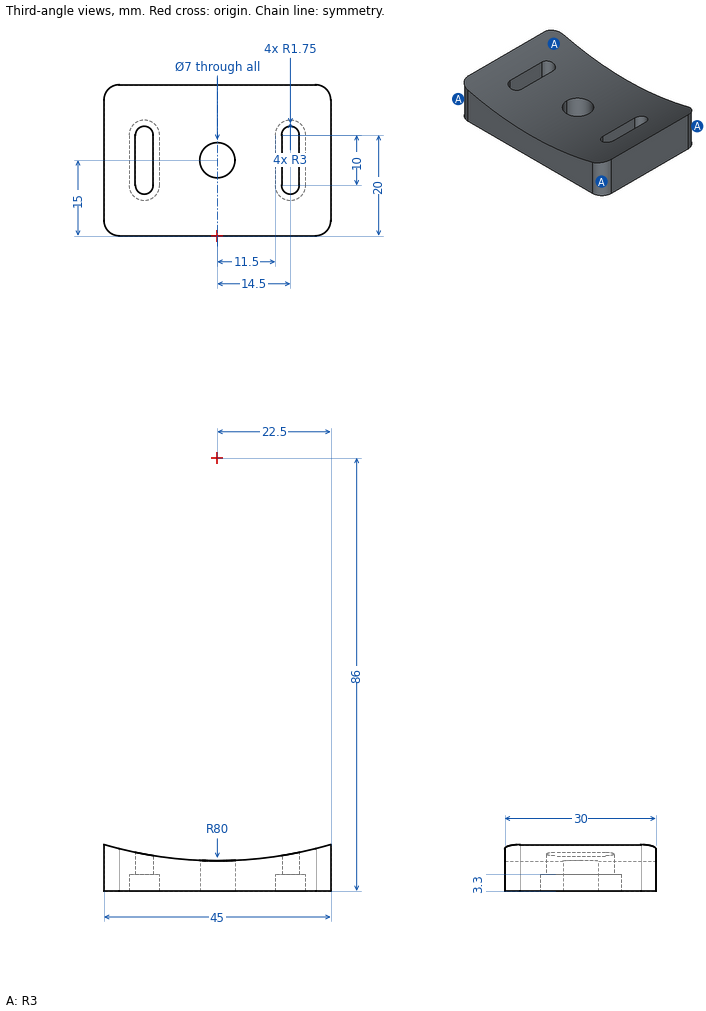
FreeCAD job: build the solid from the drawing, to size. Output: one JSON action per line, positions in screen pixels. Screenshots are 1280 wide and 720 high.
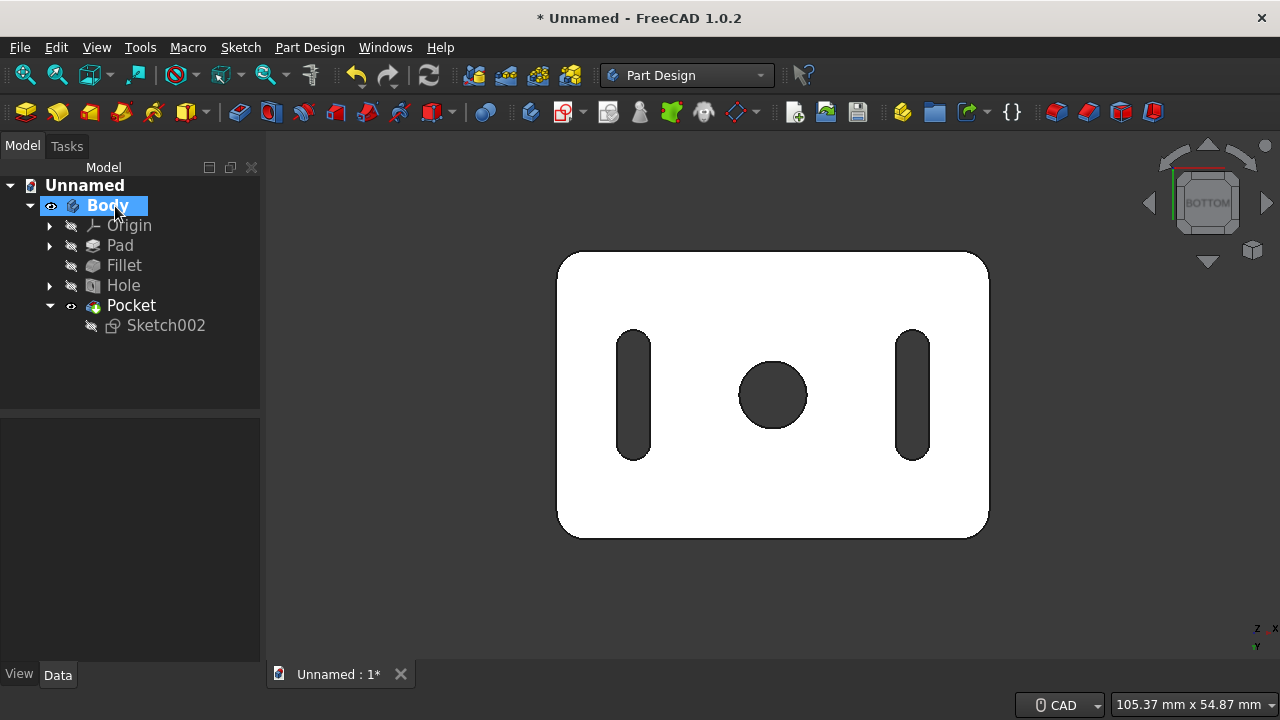
{"action": "left_click", "coordinate": [835, 476]}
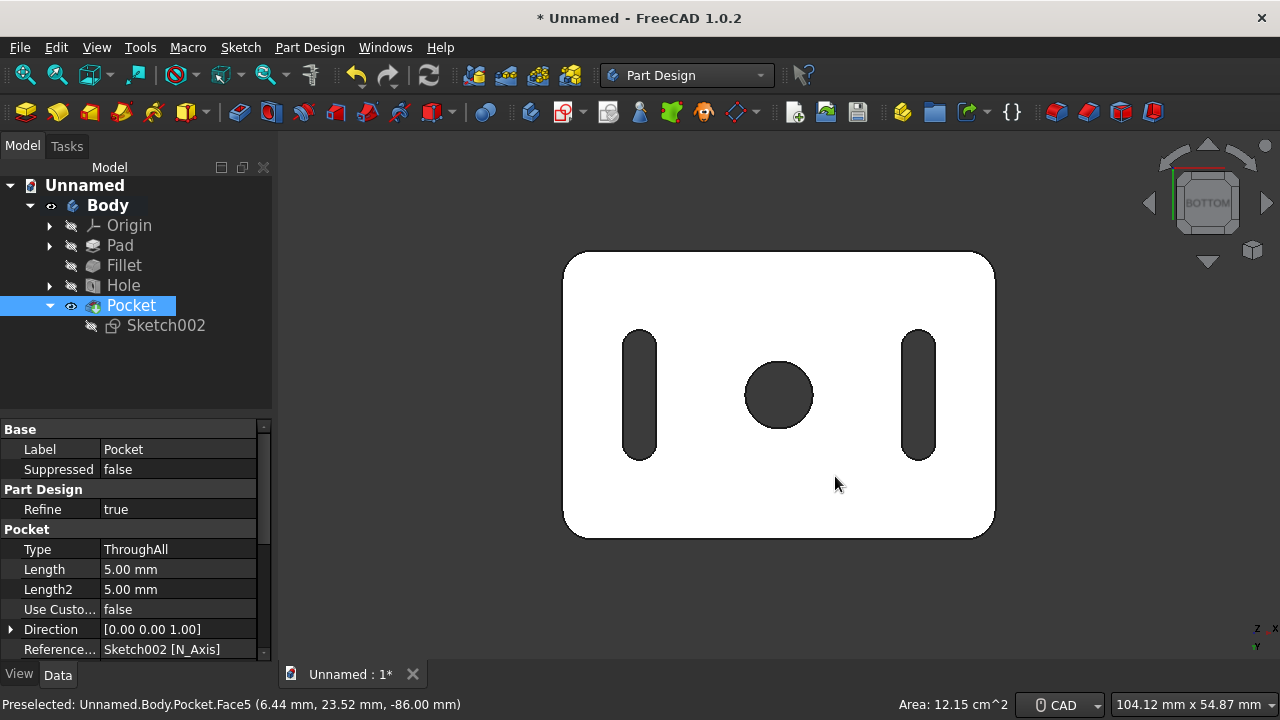
{"action": "left_click", "coordinate": [564, 112]}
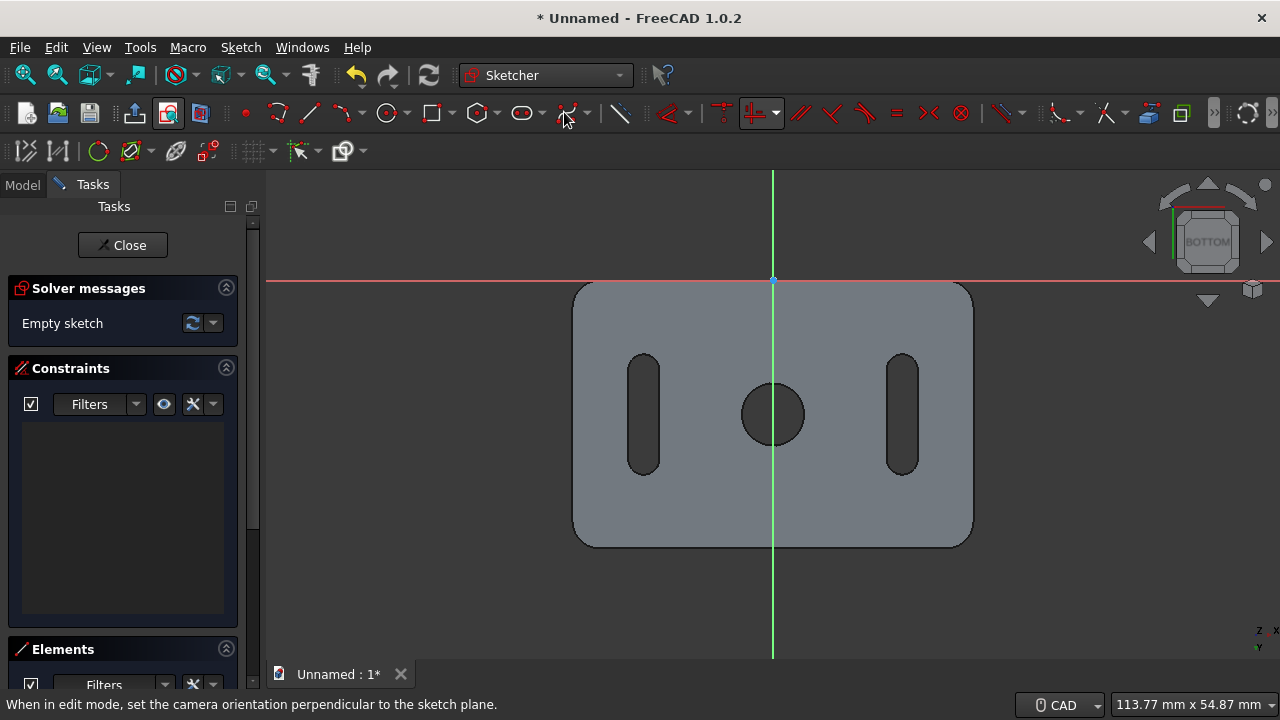
{"action": "scroll", "coordinate": [912, 320], "scroll_direction": "up", "scroll_amount": 2}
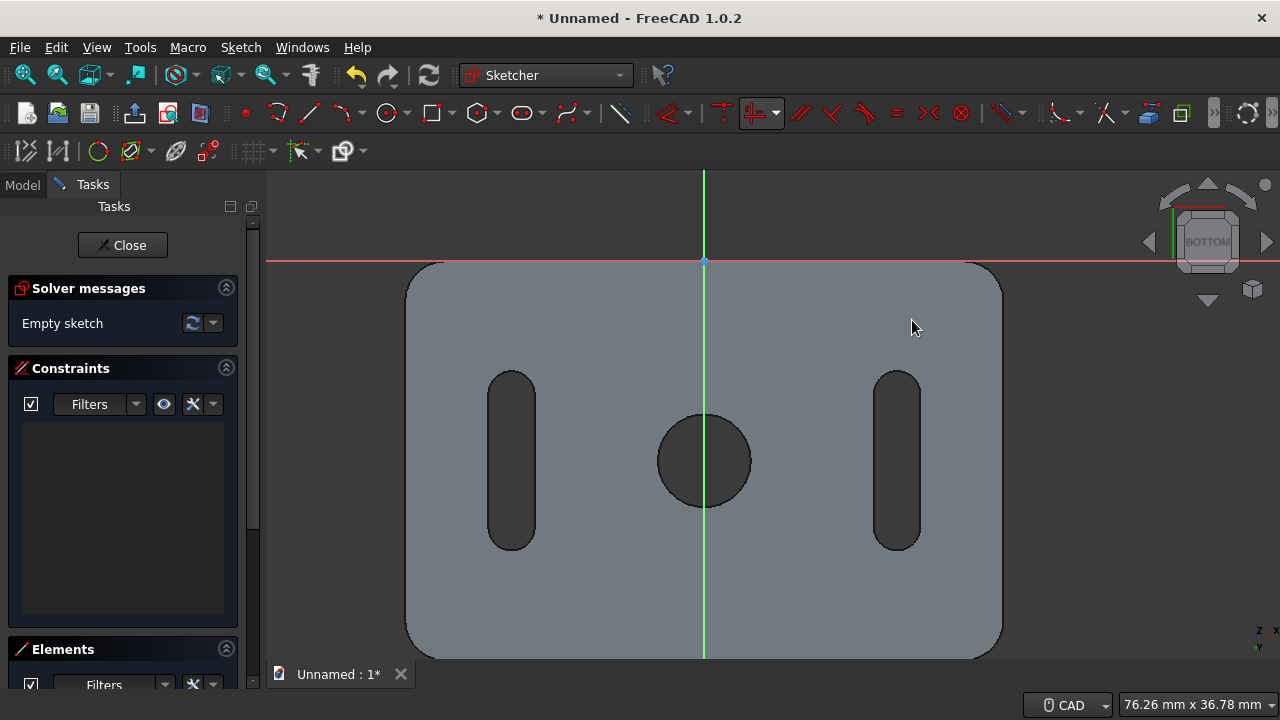
{"action": "key", "text": "g s"}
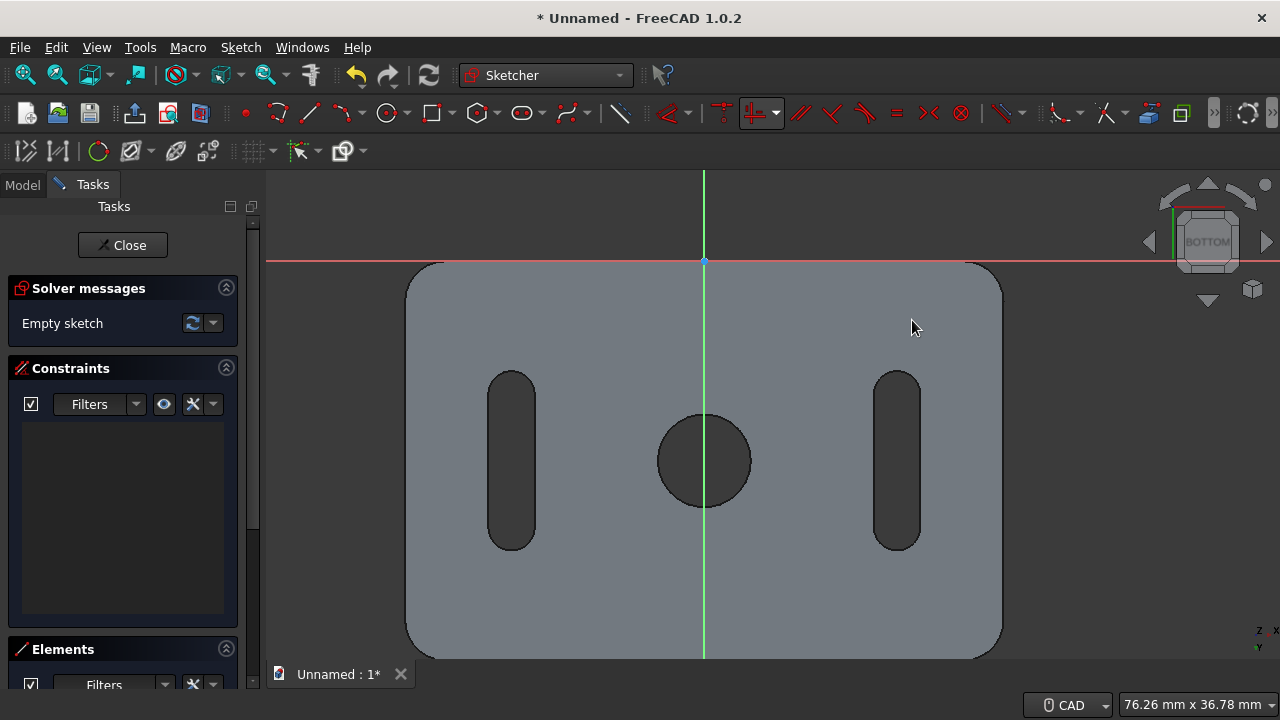
{"action": "left_click", "coordinate": [897, 527]}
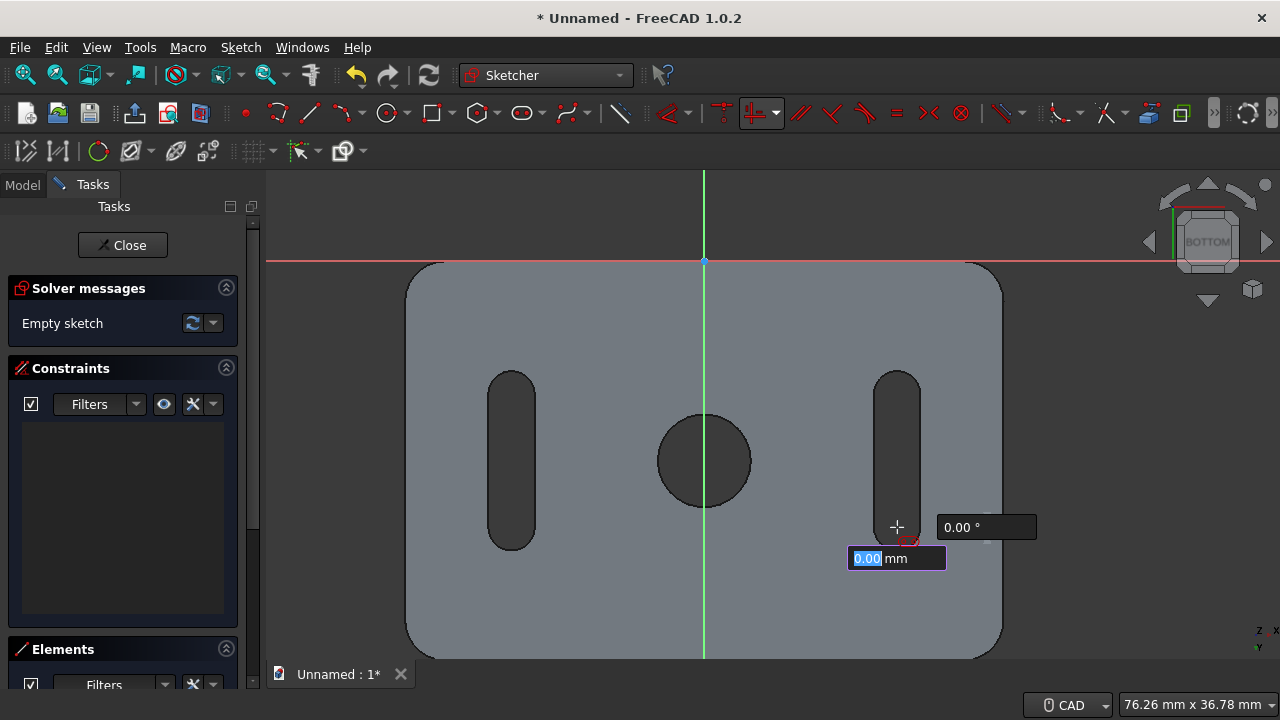
{"action": "left_click", "coordinate": [897, 394]}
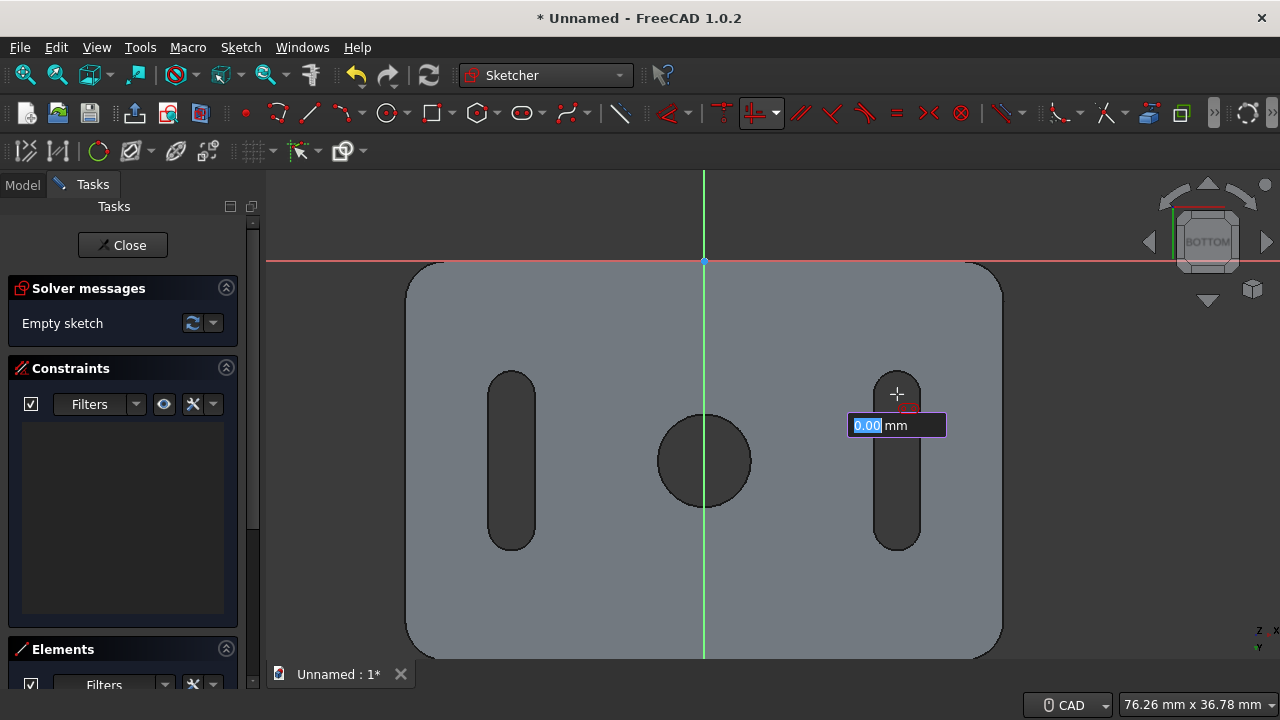
{"action": "left_click", "coordinate": [857, 461]}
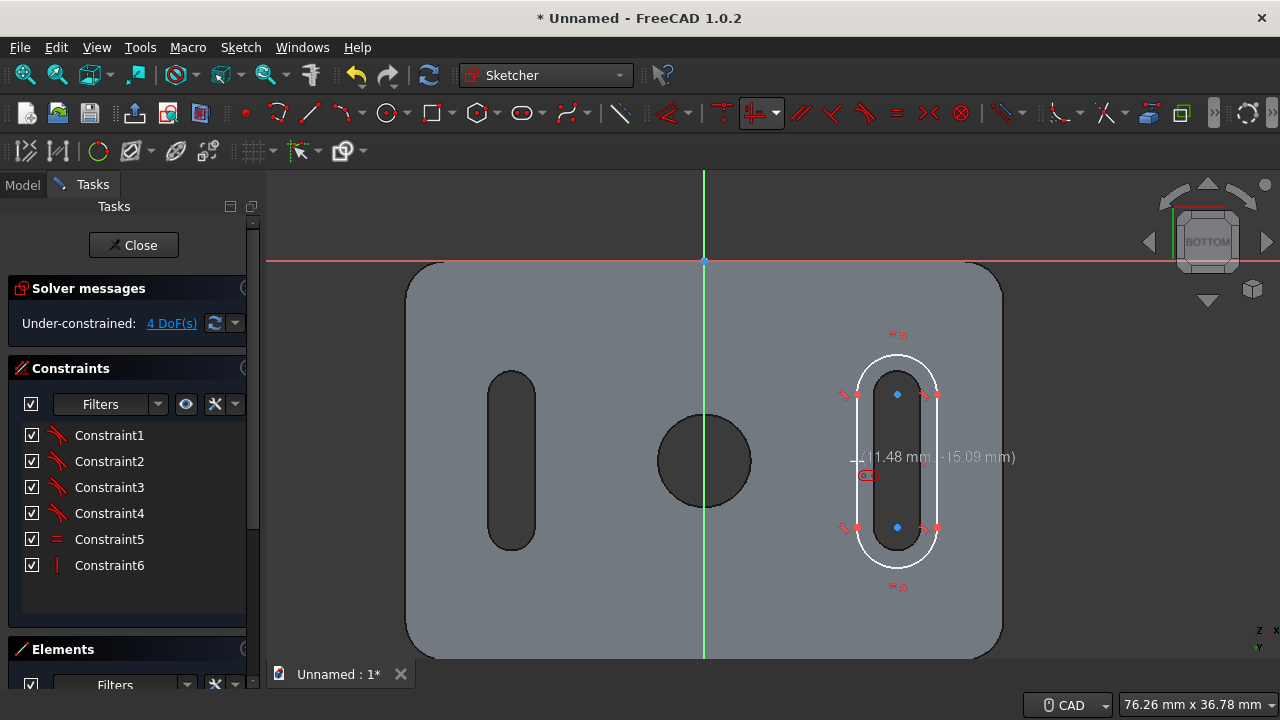
{"action": "left_click", "coordinate": [512, 527]}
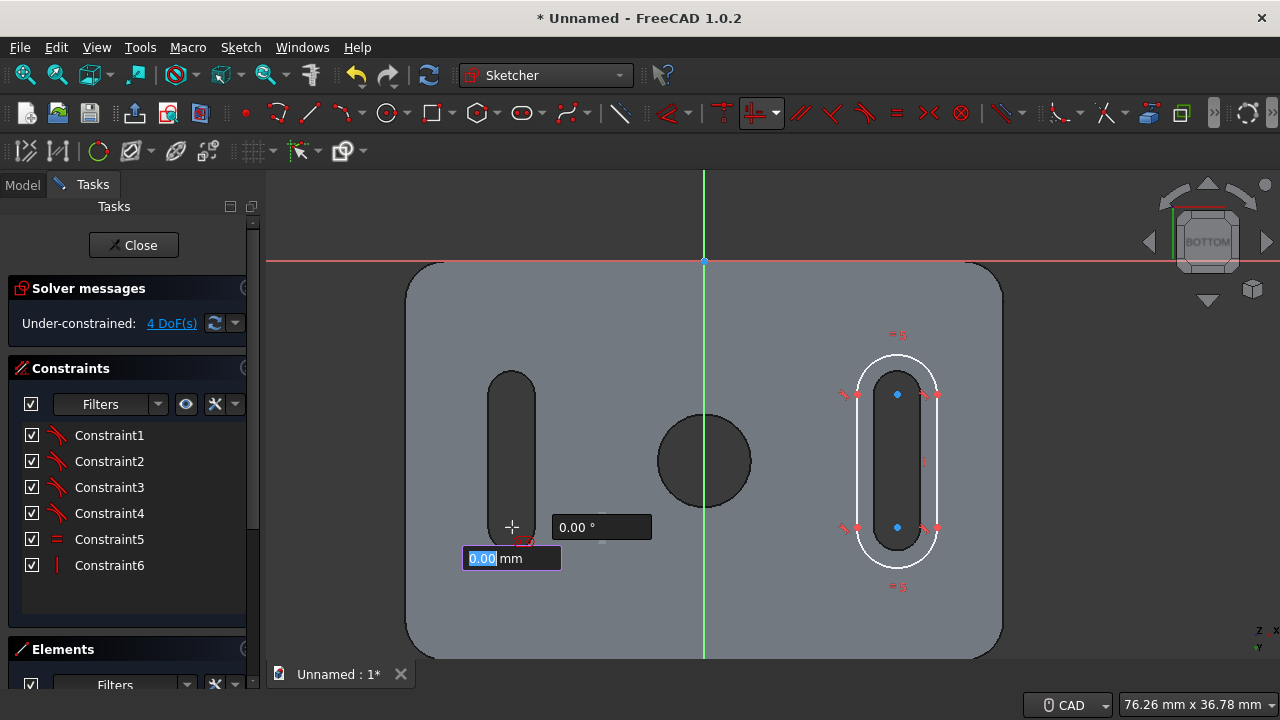
{"action": "left_click", "coordinate": [512, 394]}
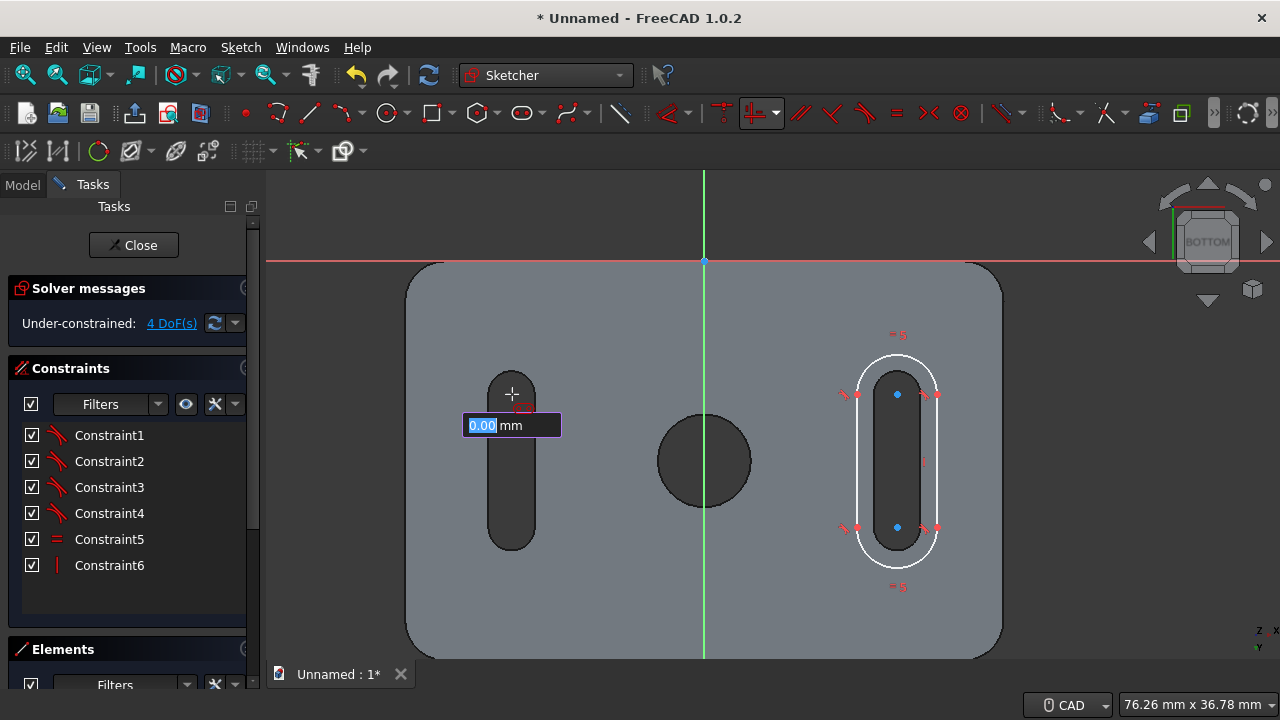
{"action": "left_click", "coordinate": [472, 461]}
{"action": "key", "text": "Escape"}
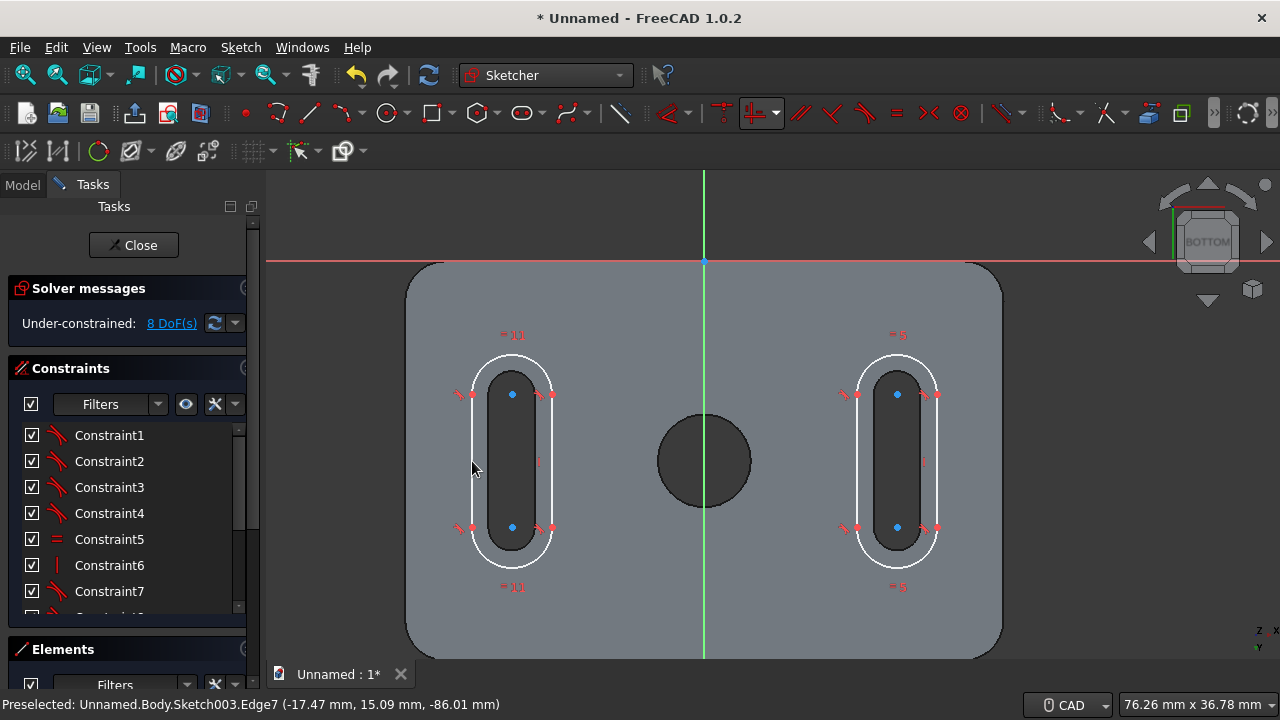
{"action": "left_click", "coordinate": [873, 560]}